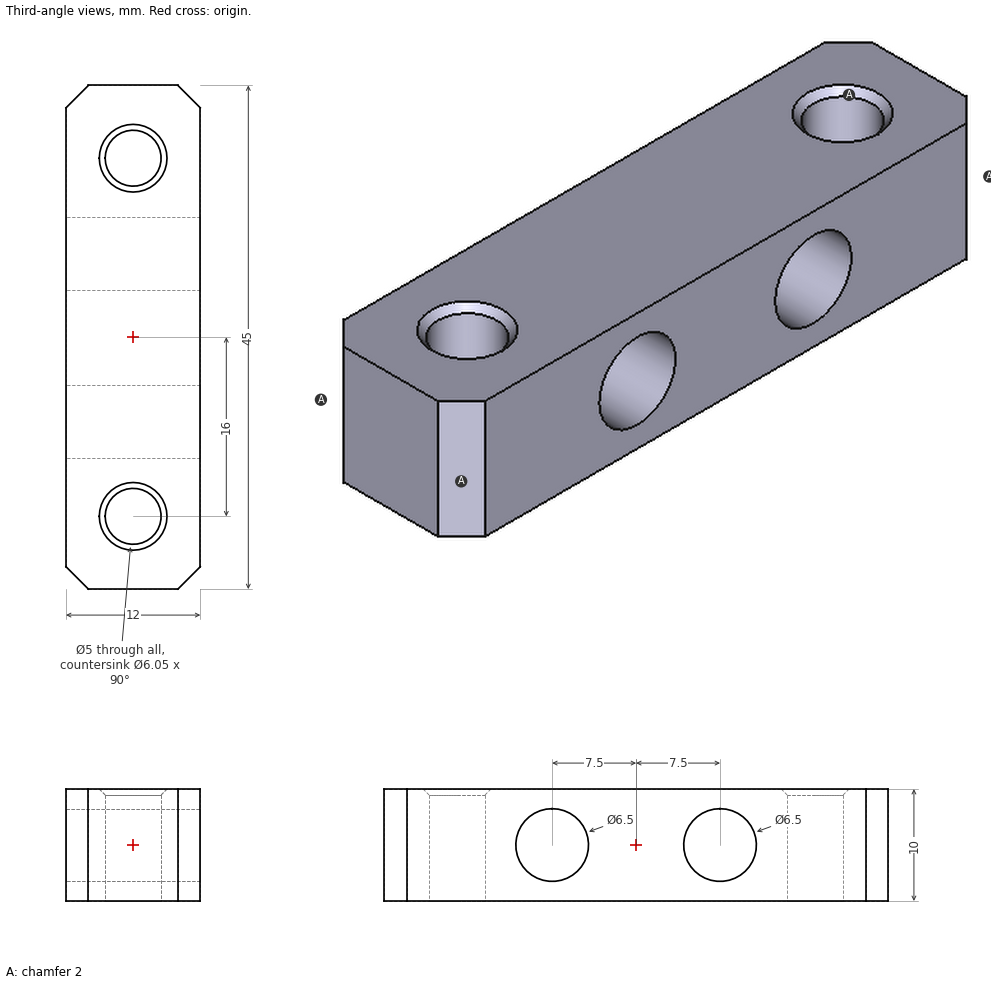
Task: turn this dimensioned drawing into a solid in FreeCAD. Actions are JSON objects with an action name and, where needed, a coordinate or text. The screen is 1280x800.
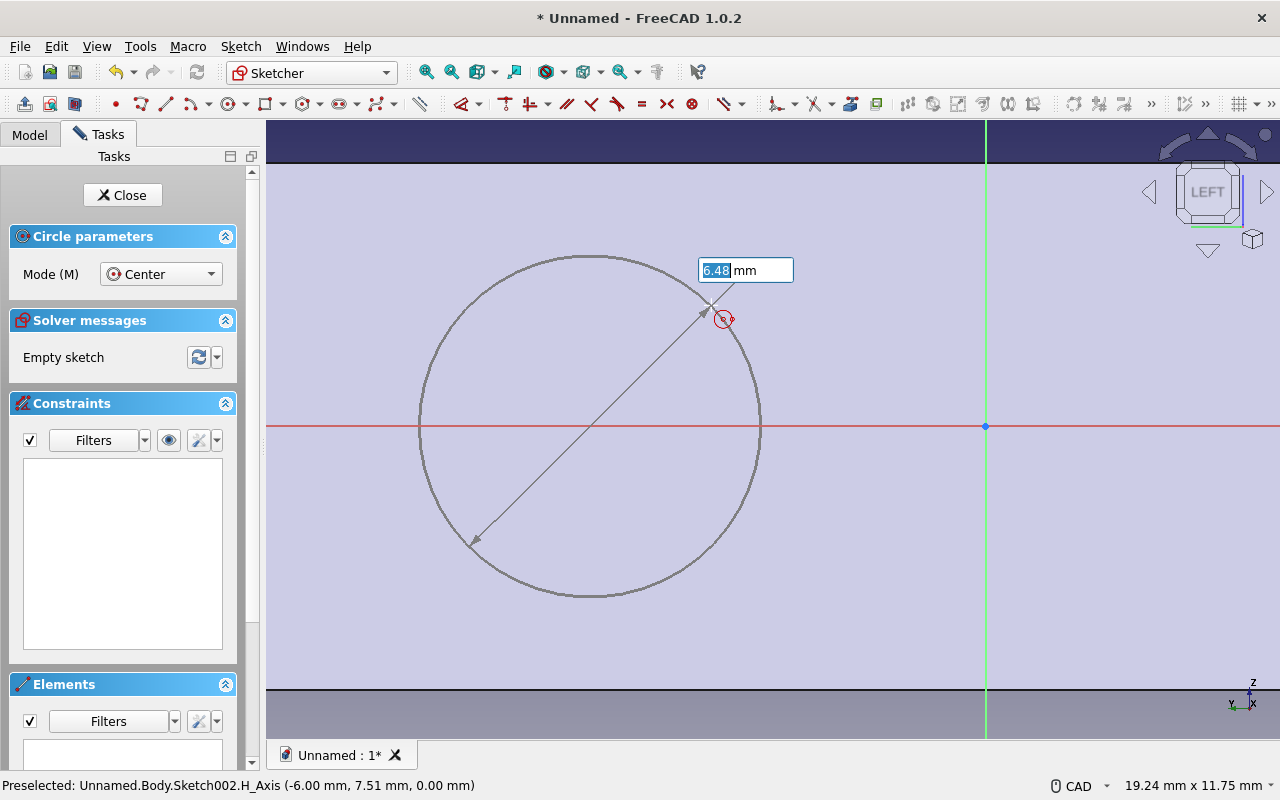
{"action": "type", "text": "6.5"}
{"action": "key", "text": "Return"}
{"action": "key", "text": "Escape"}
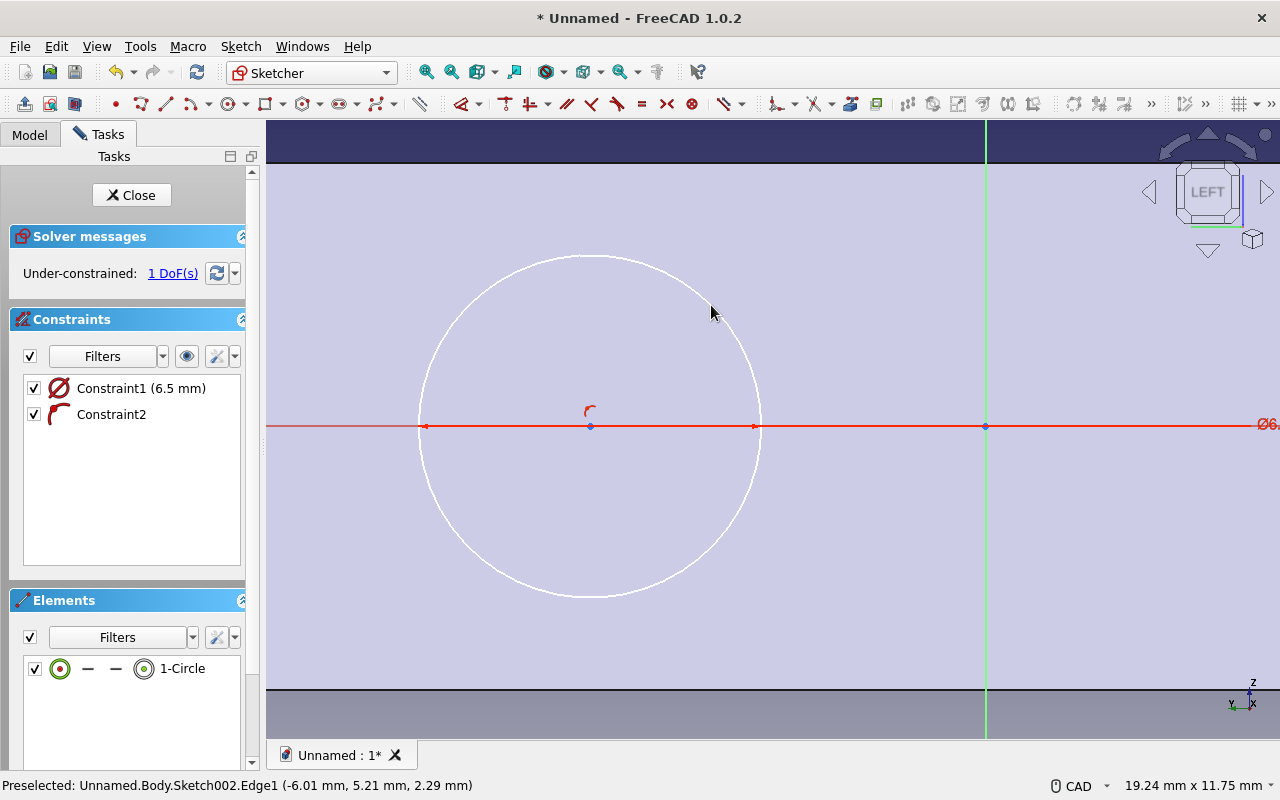
{"action": "left_click", "coordinate": [460, 104]}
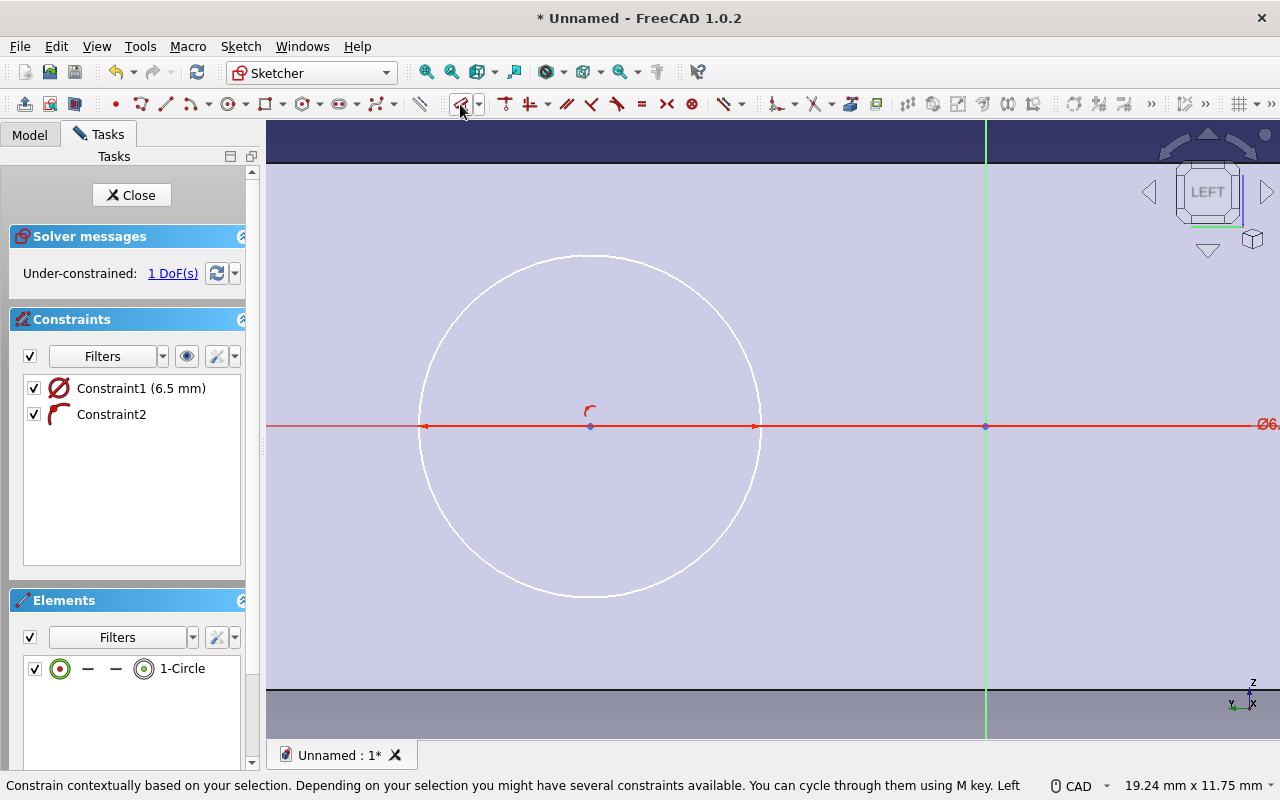
{"action": "left_click", "coordinate": [590, 426]}
{"action": "left_click", "coordinate": [788, 460]}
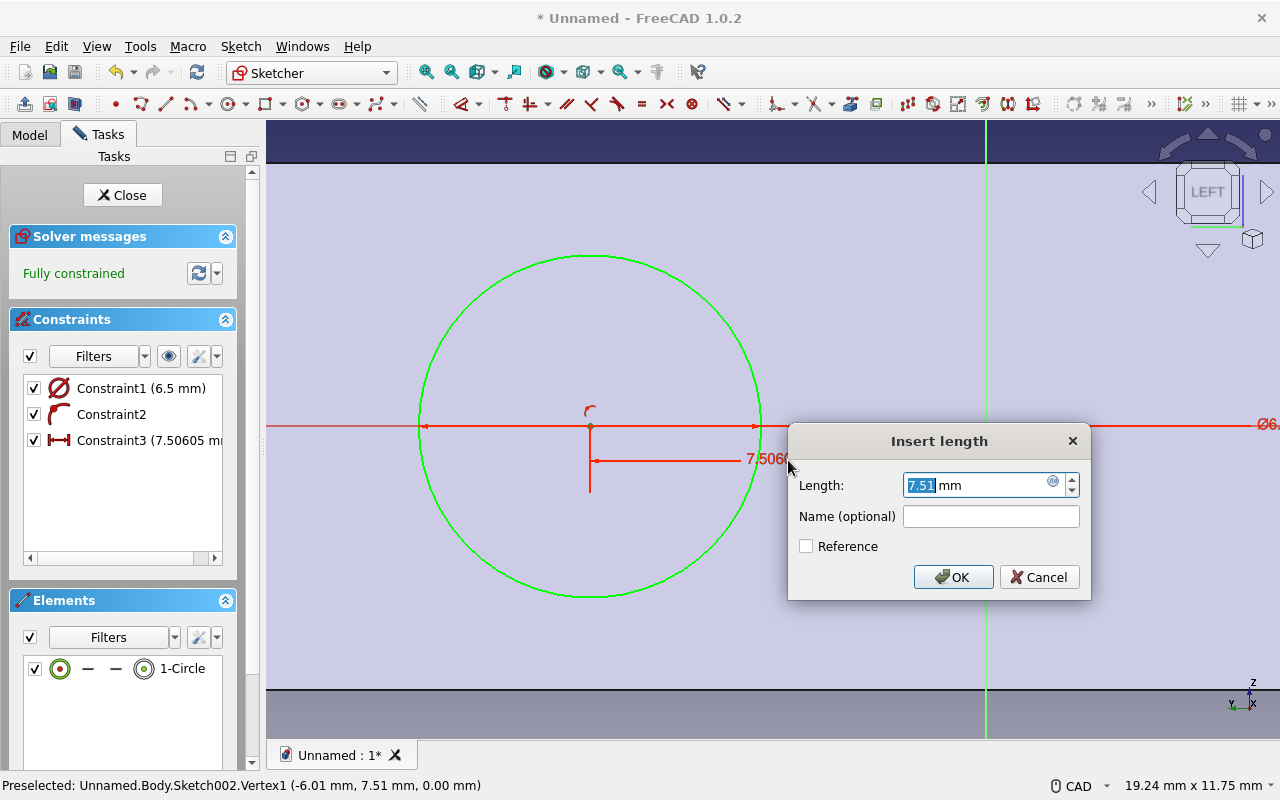
{"action": "type", "text": "7.5"}
{"action": "key", "text": "Return"}
{"action": "key", "text": "Escape"}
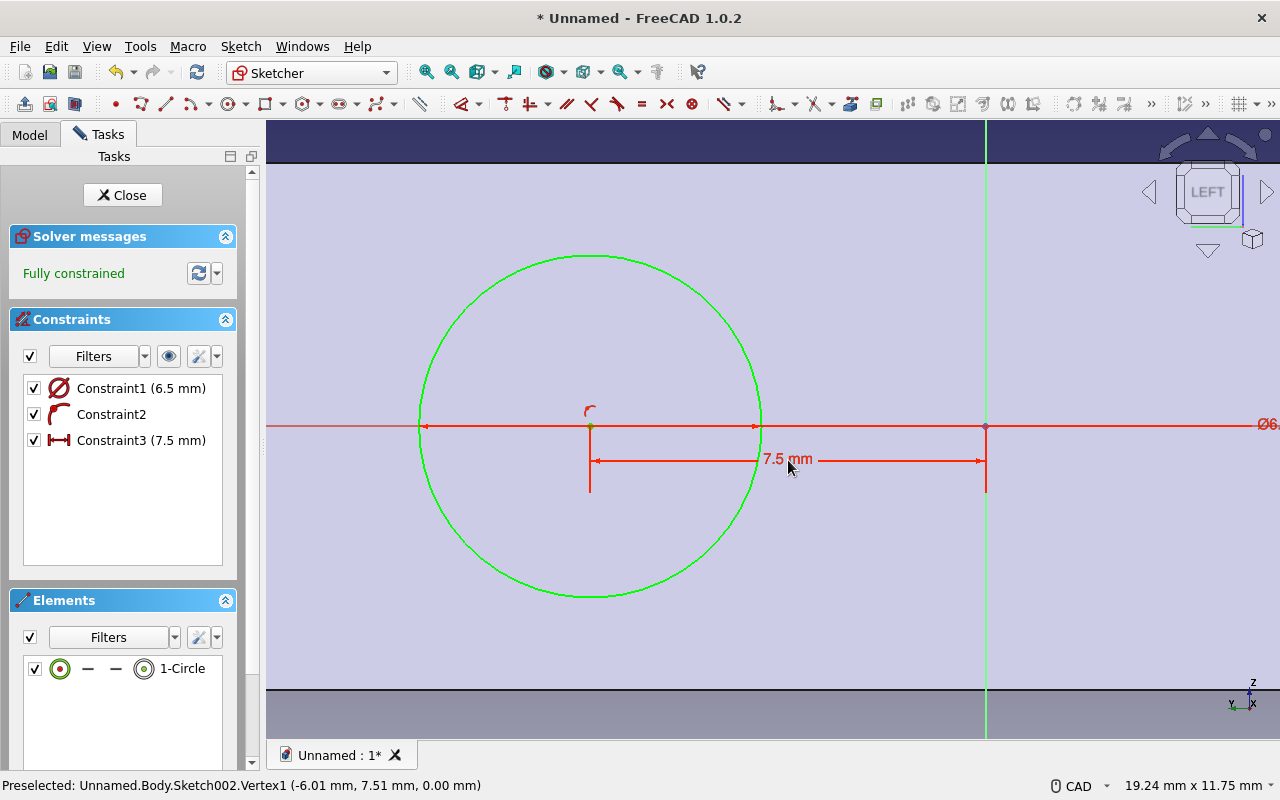
{"action": "left_click", "coordinate": [123, 195]}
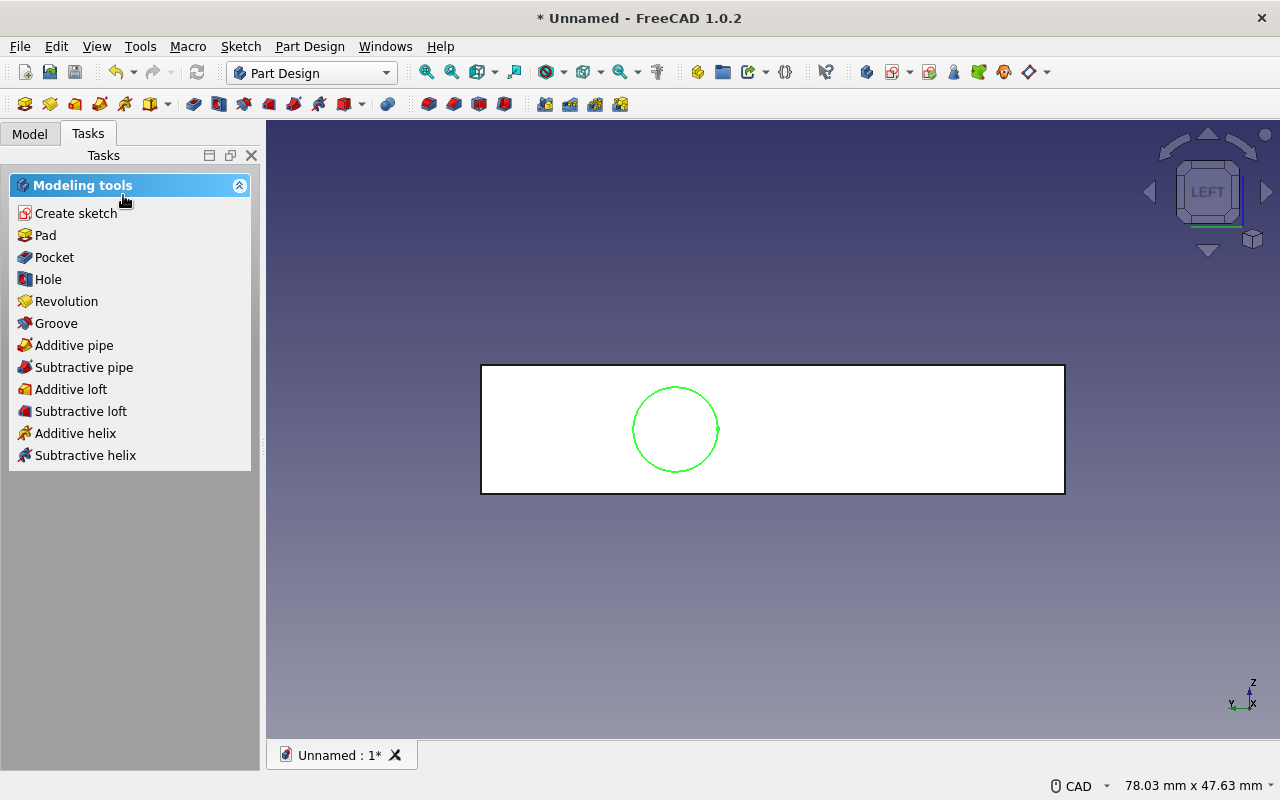
{"action": "left_click", "coordinate": [194, 104]}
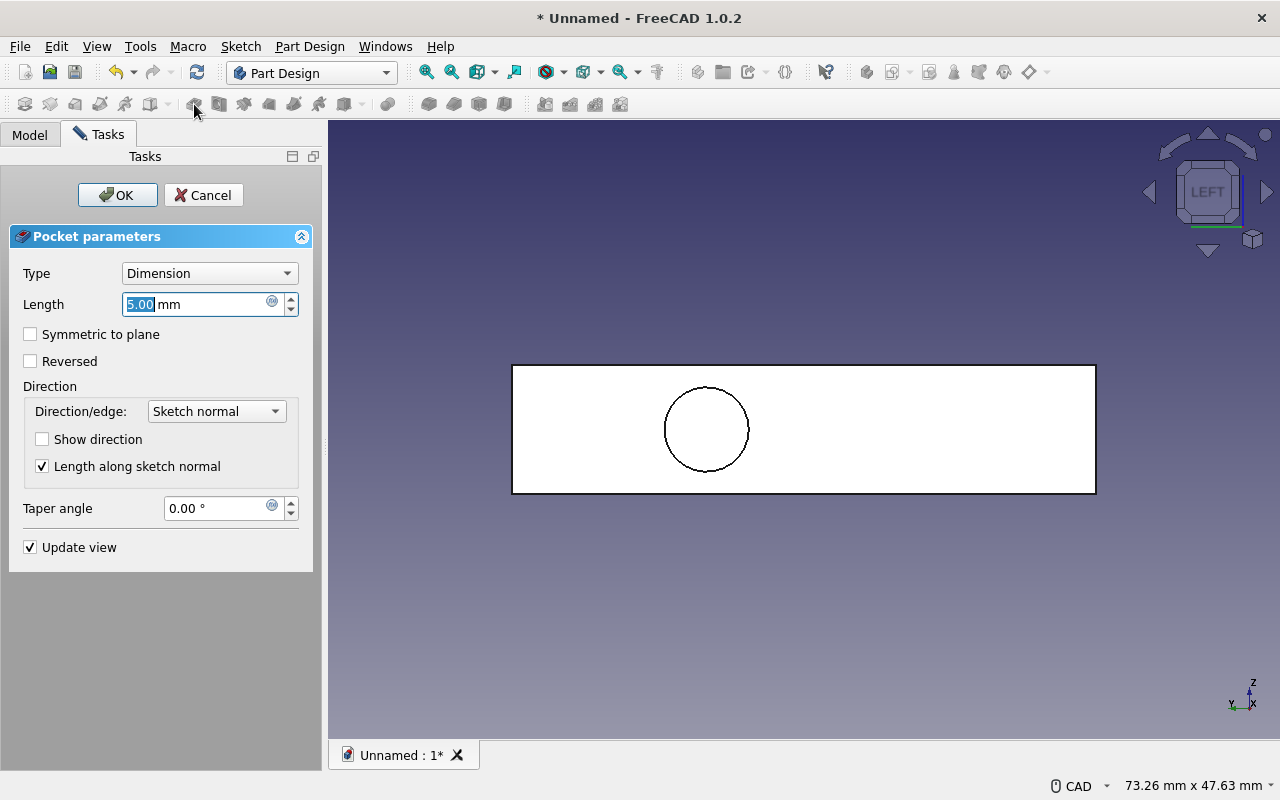
{"action": "left_click", "coordinate": [210, 274]}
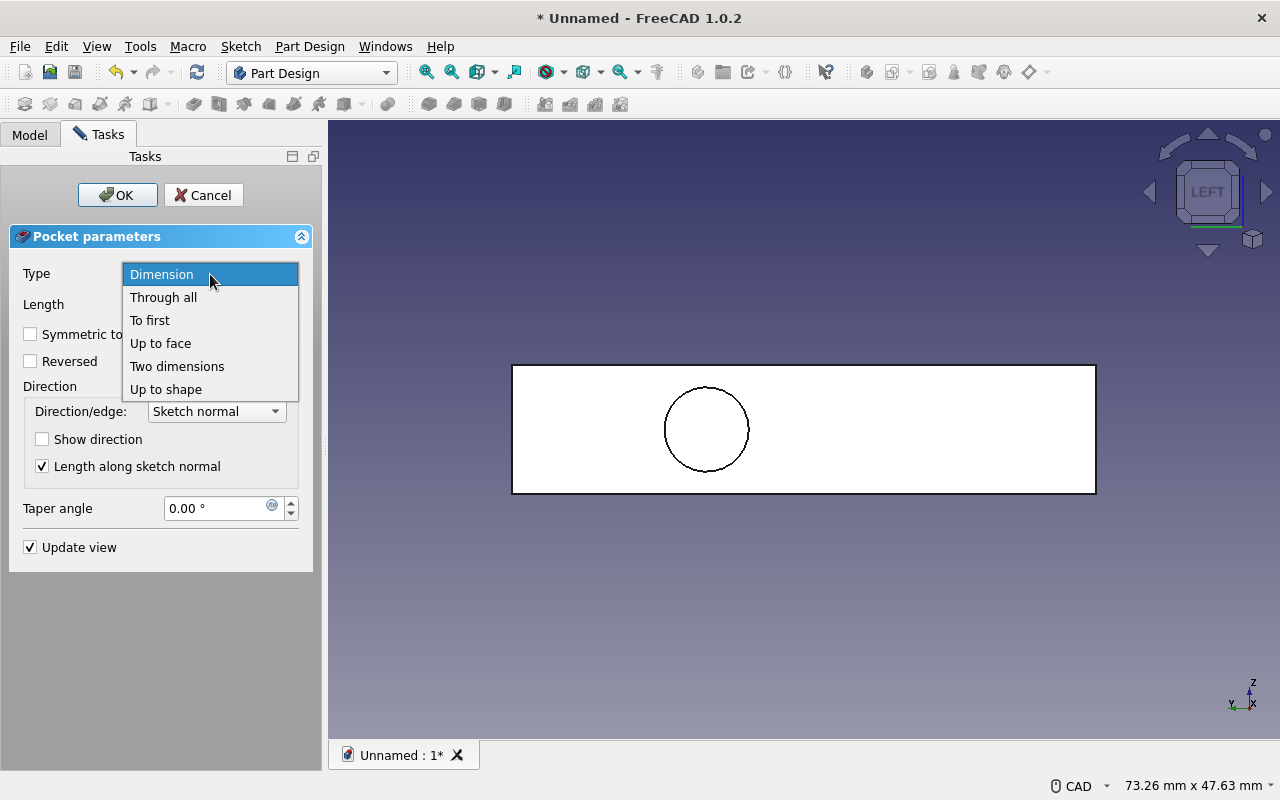
{"action": "left_click", "coordinate": [208, 320]}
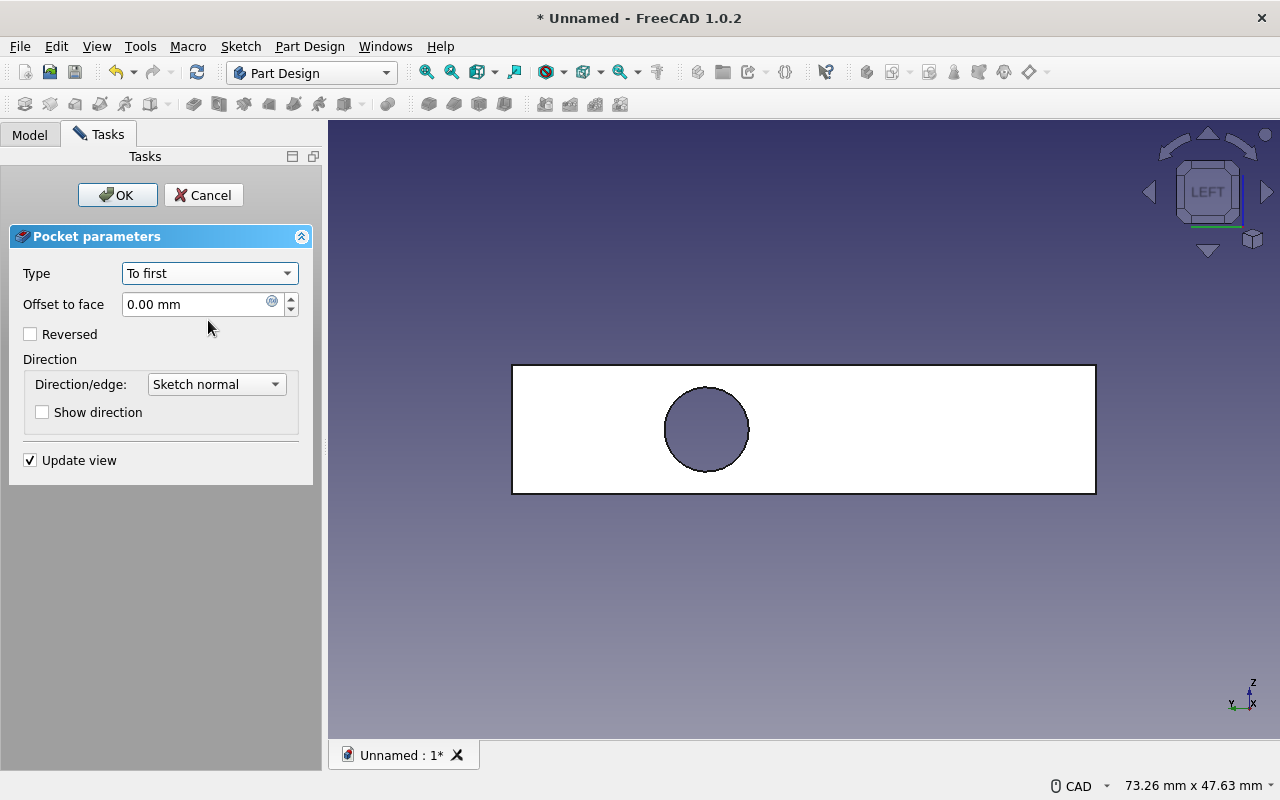
{"action": "left_click", "coordinate": [118, 195]}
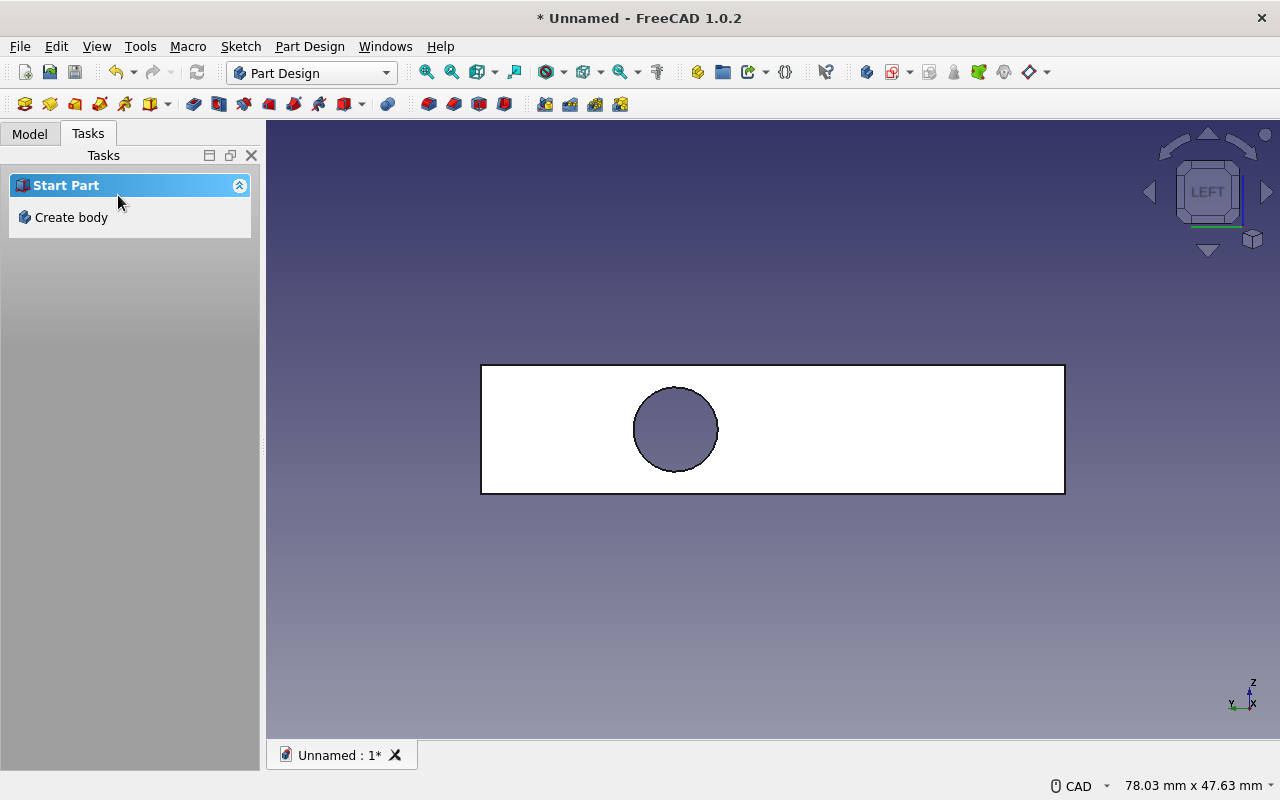
{"action": "left_click", "coordinate": [857, 428]}